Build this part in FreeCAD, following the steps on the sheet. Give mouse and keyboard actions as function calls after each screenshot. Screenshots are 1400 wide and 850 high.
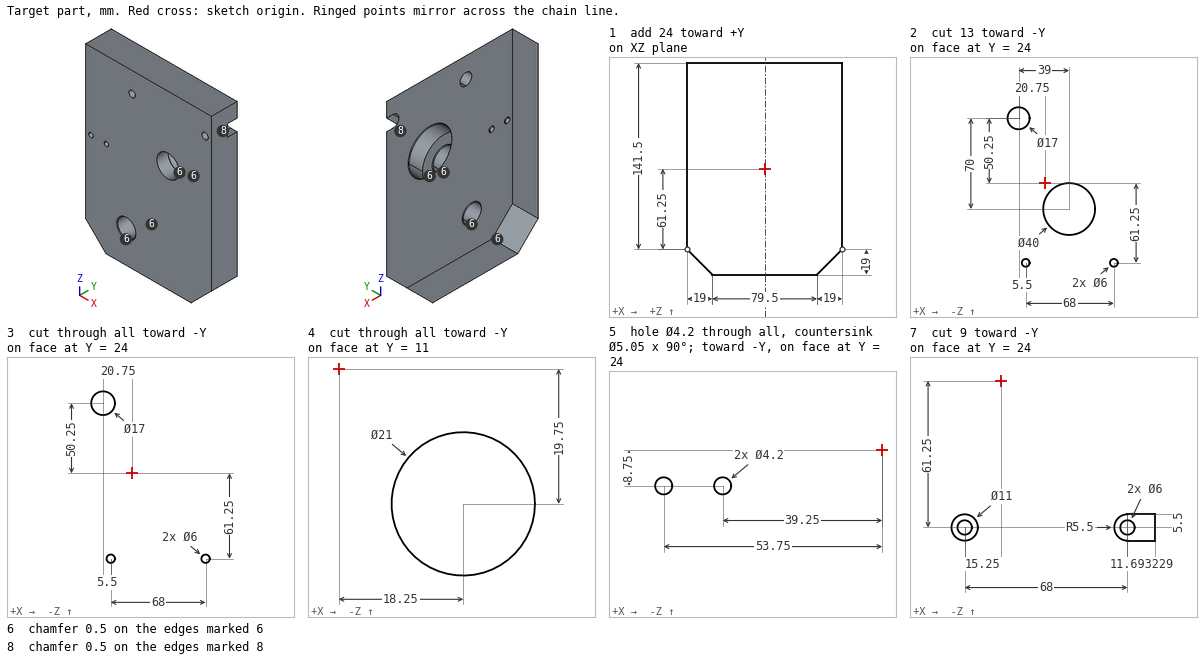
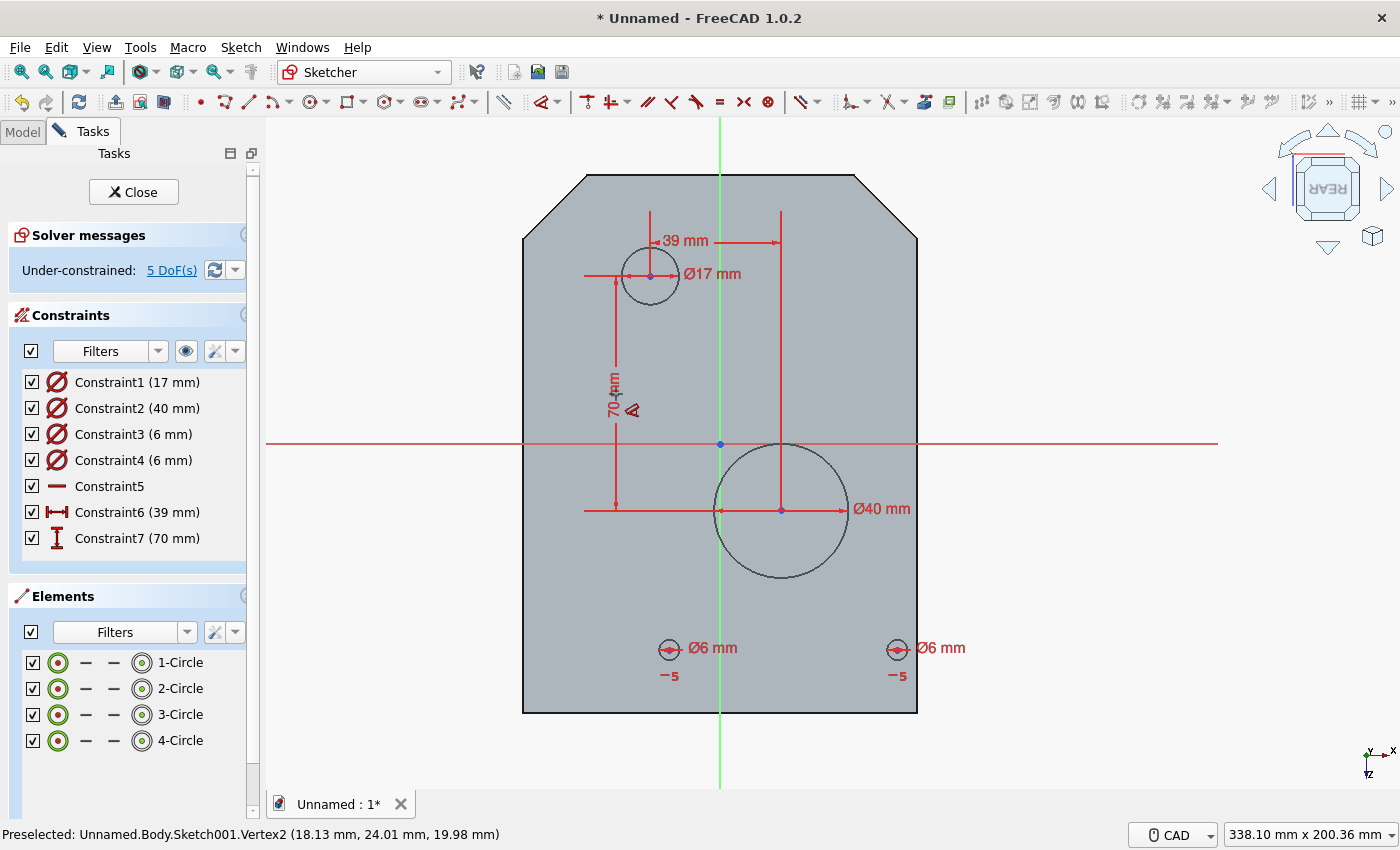
click(897, 650)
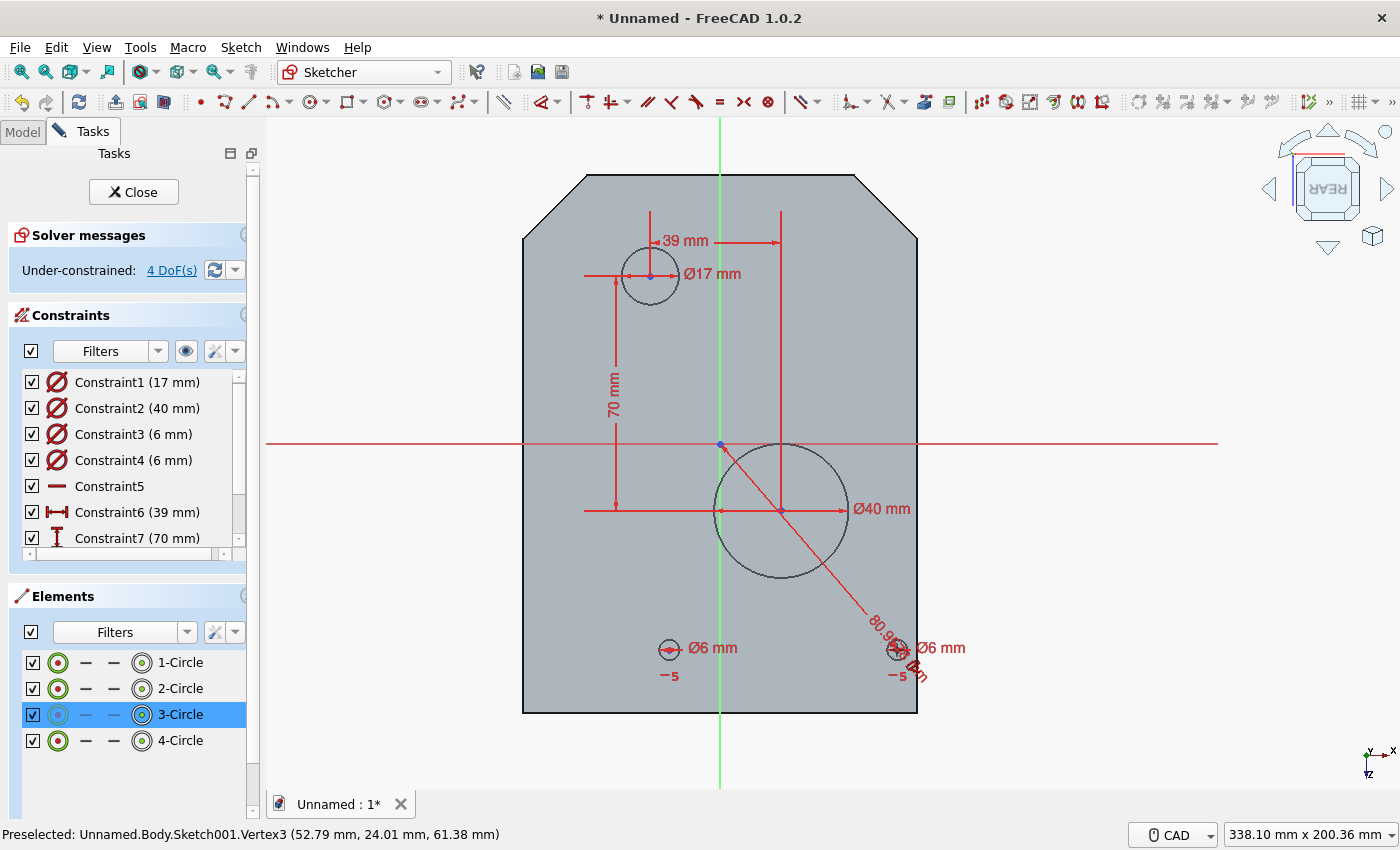
click(669, 650)
click(783, 684)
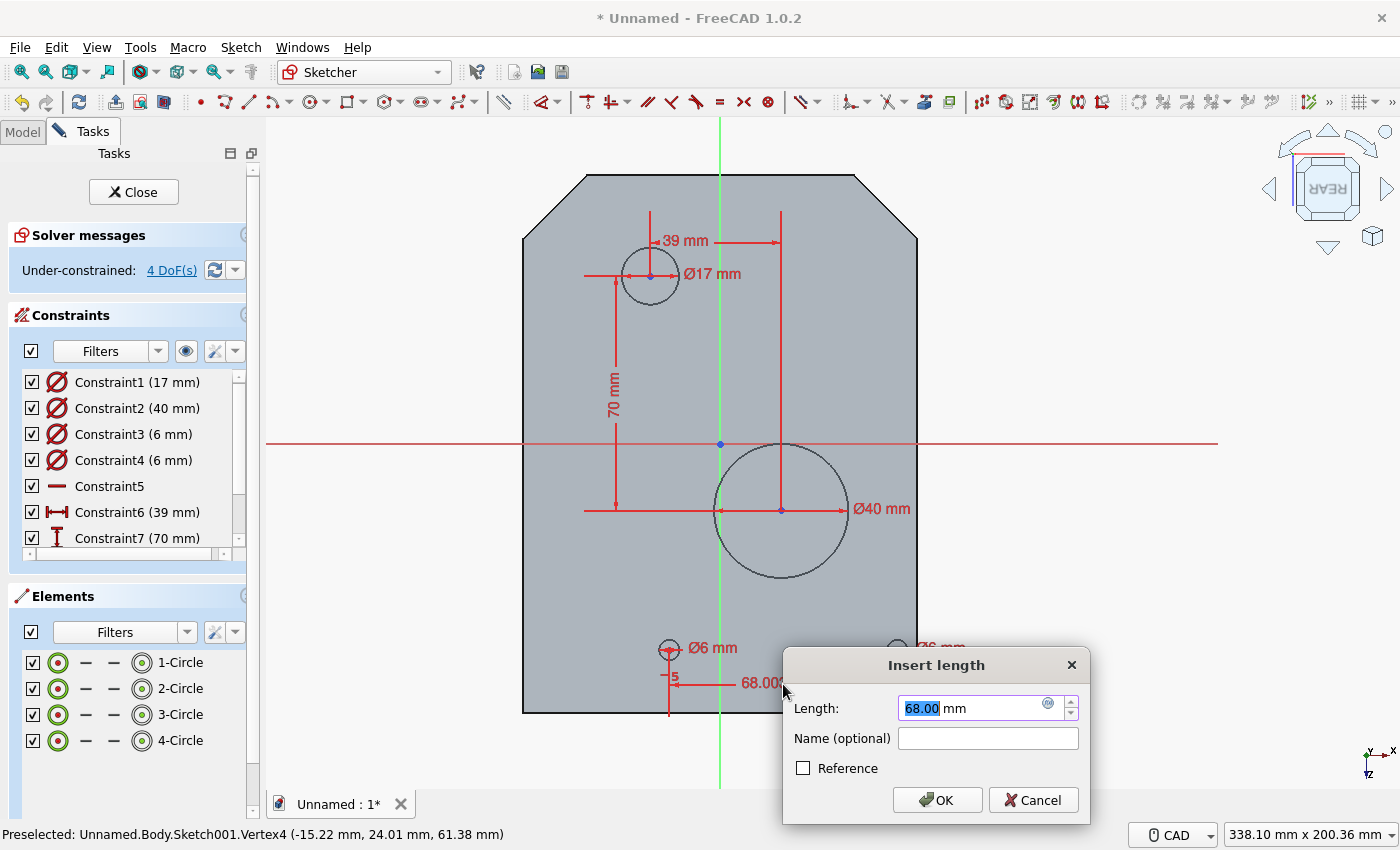
text(68)
key(Return)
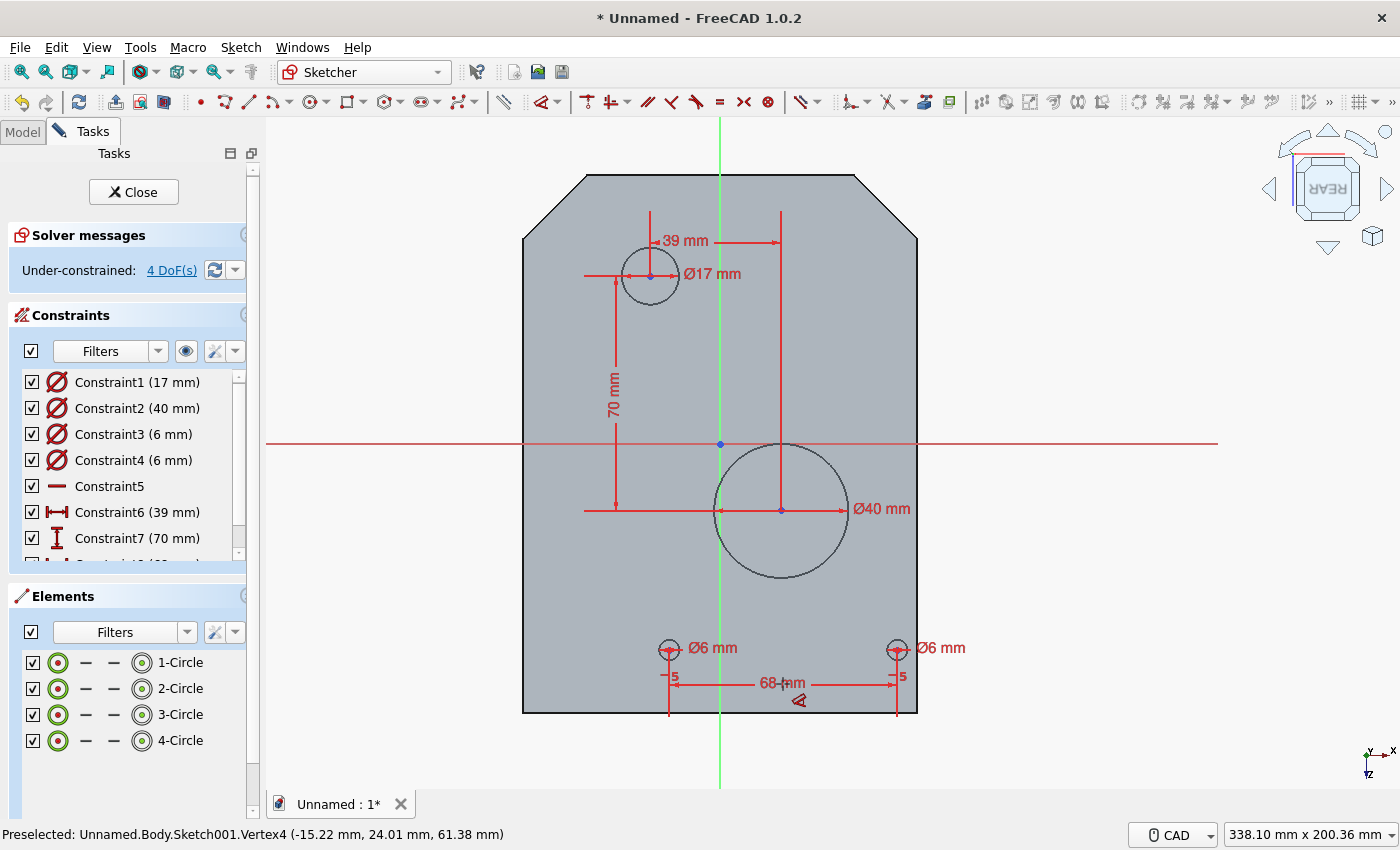
scroll(650, 276, up, 4)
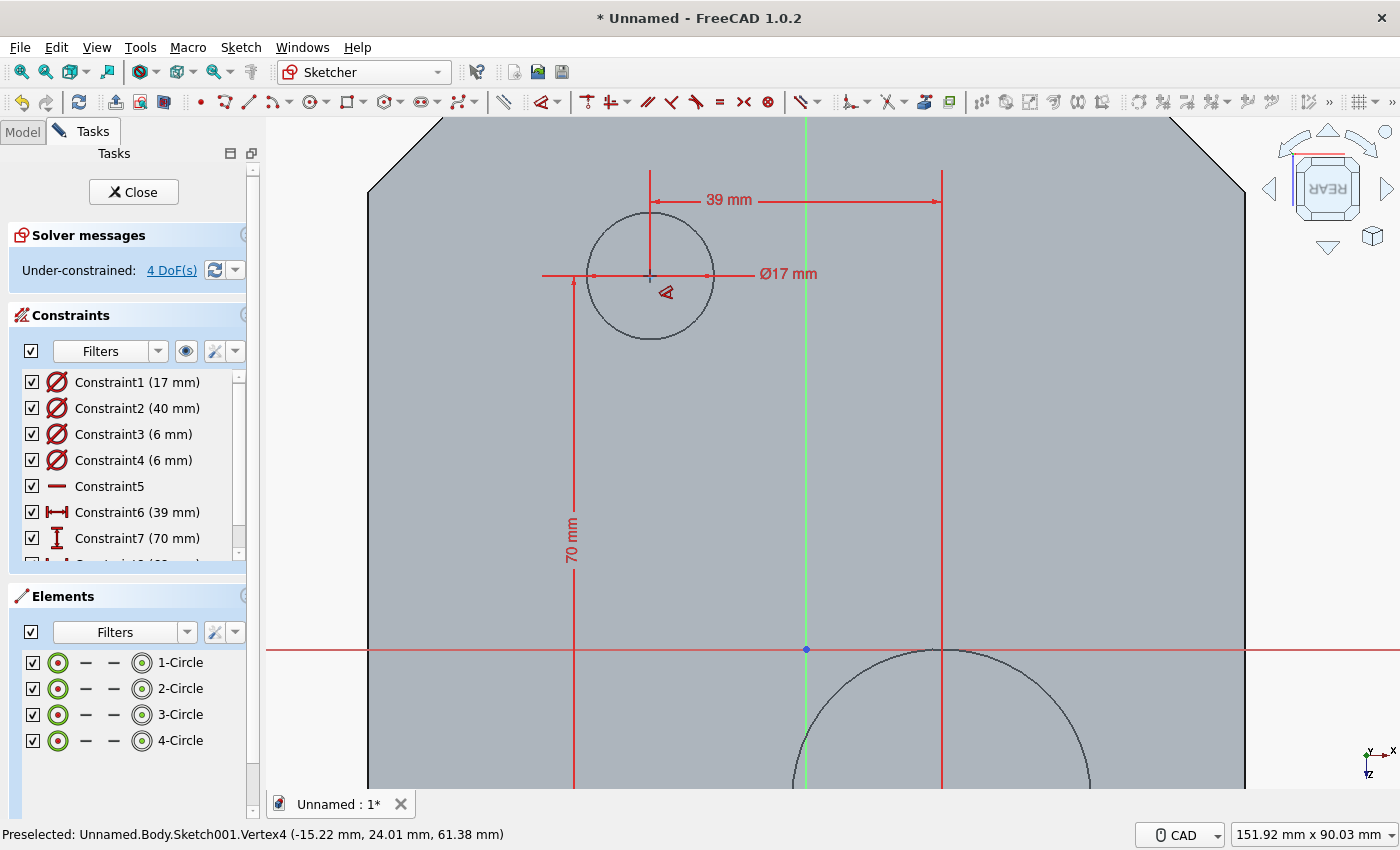
click(650, 276)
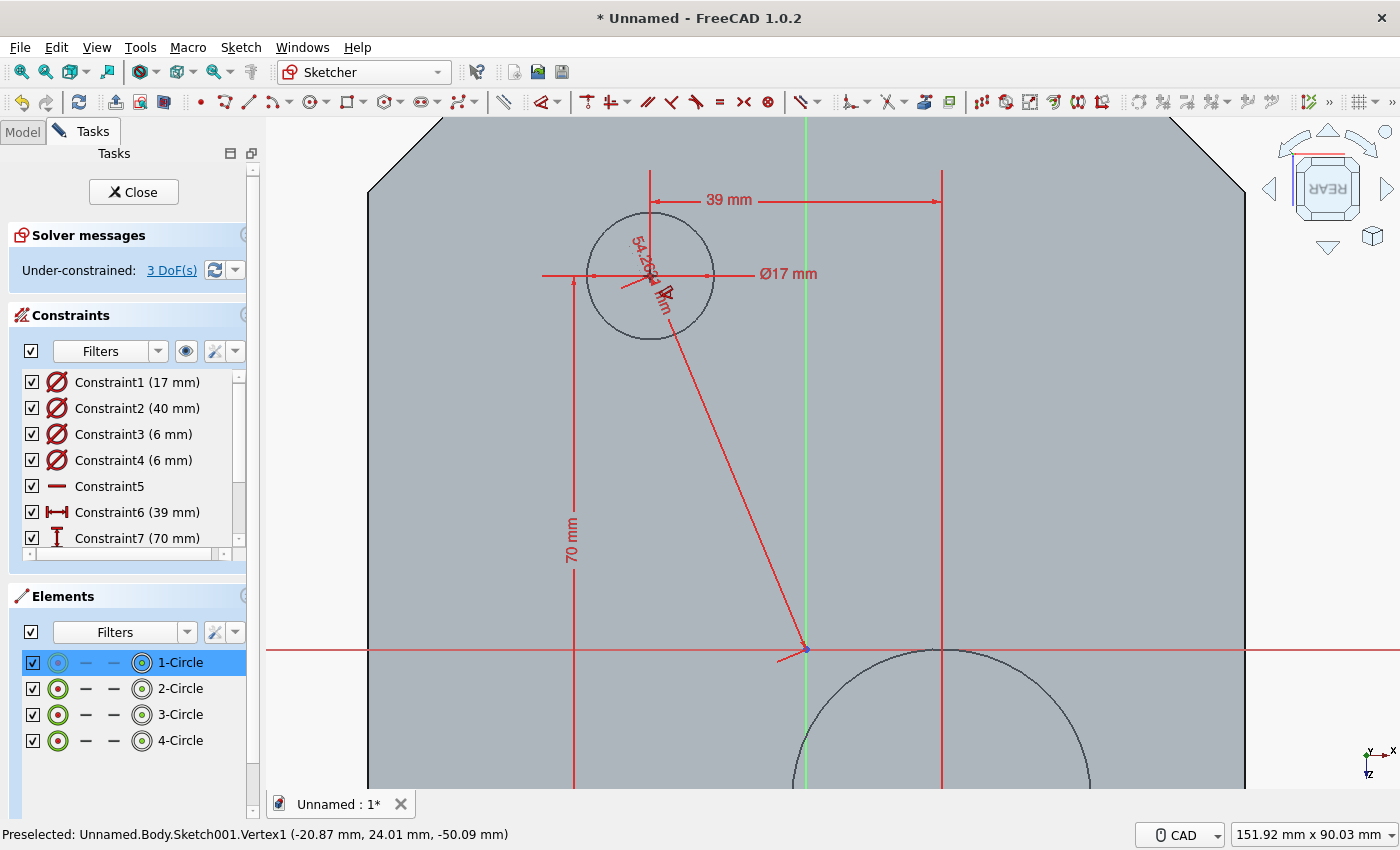
scroll(650, 276, down, 4)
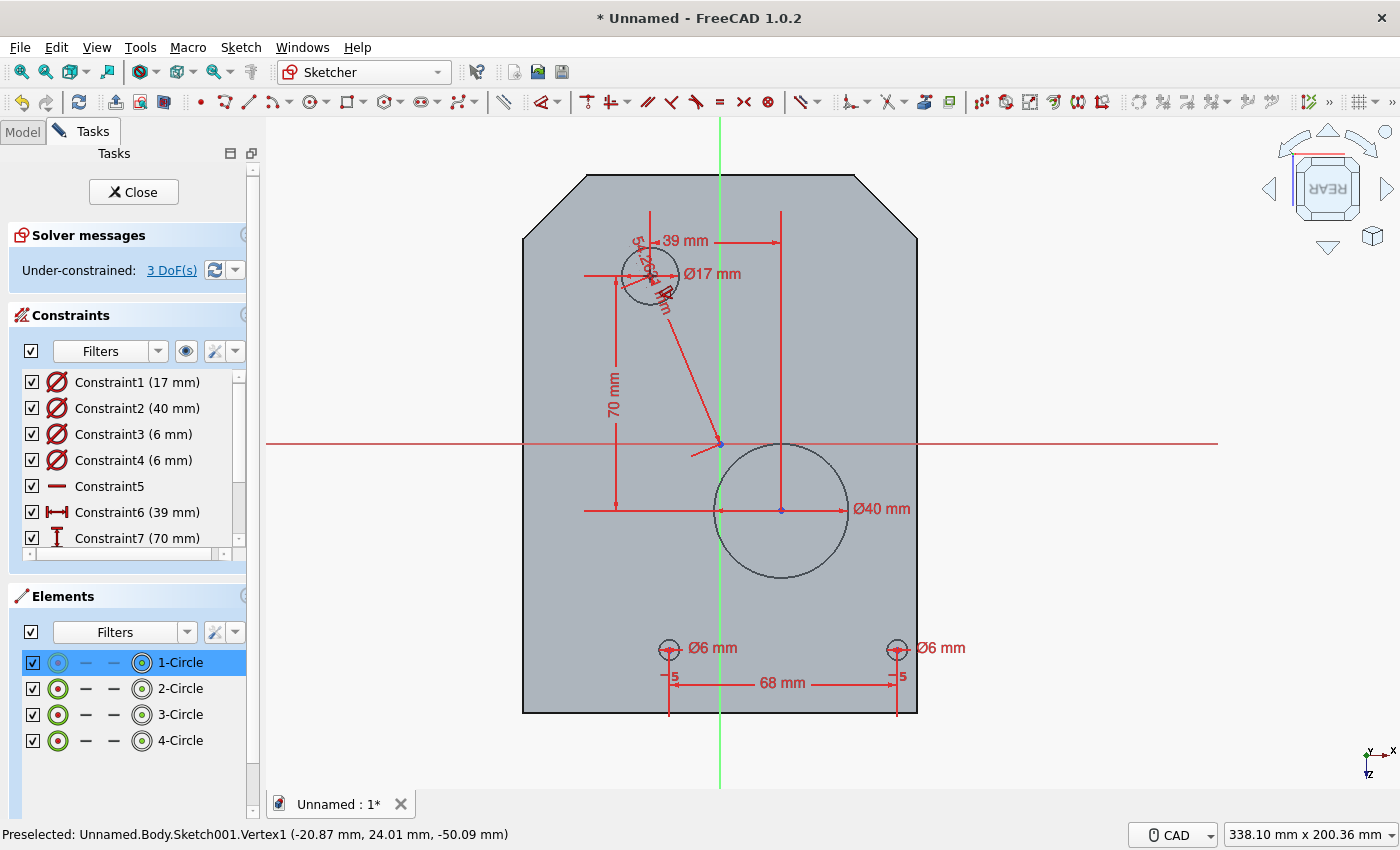
scroll(669, 650, up, 4)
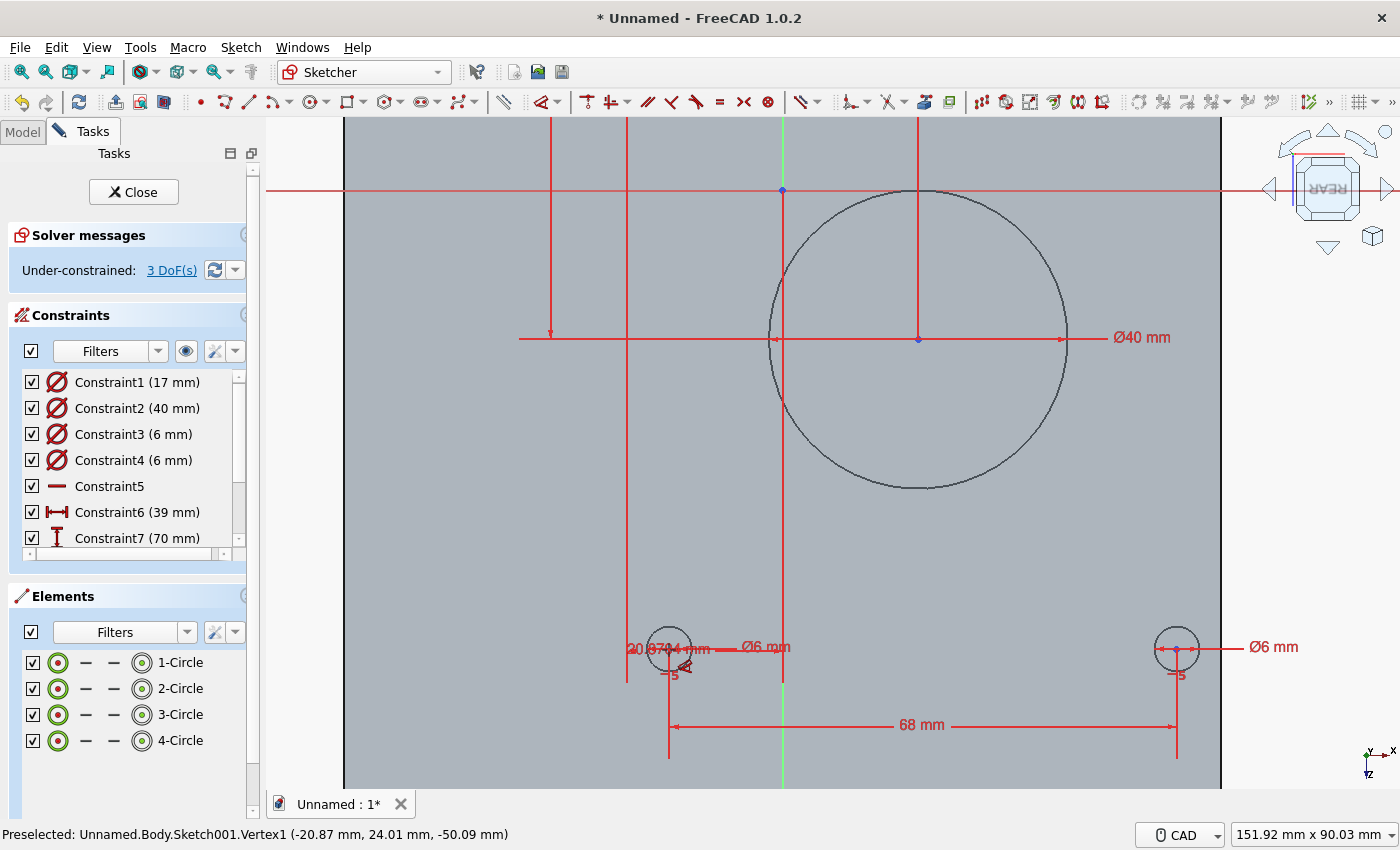
click(669, 649)
click(648, 683)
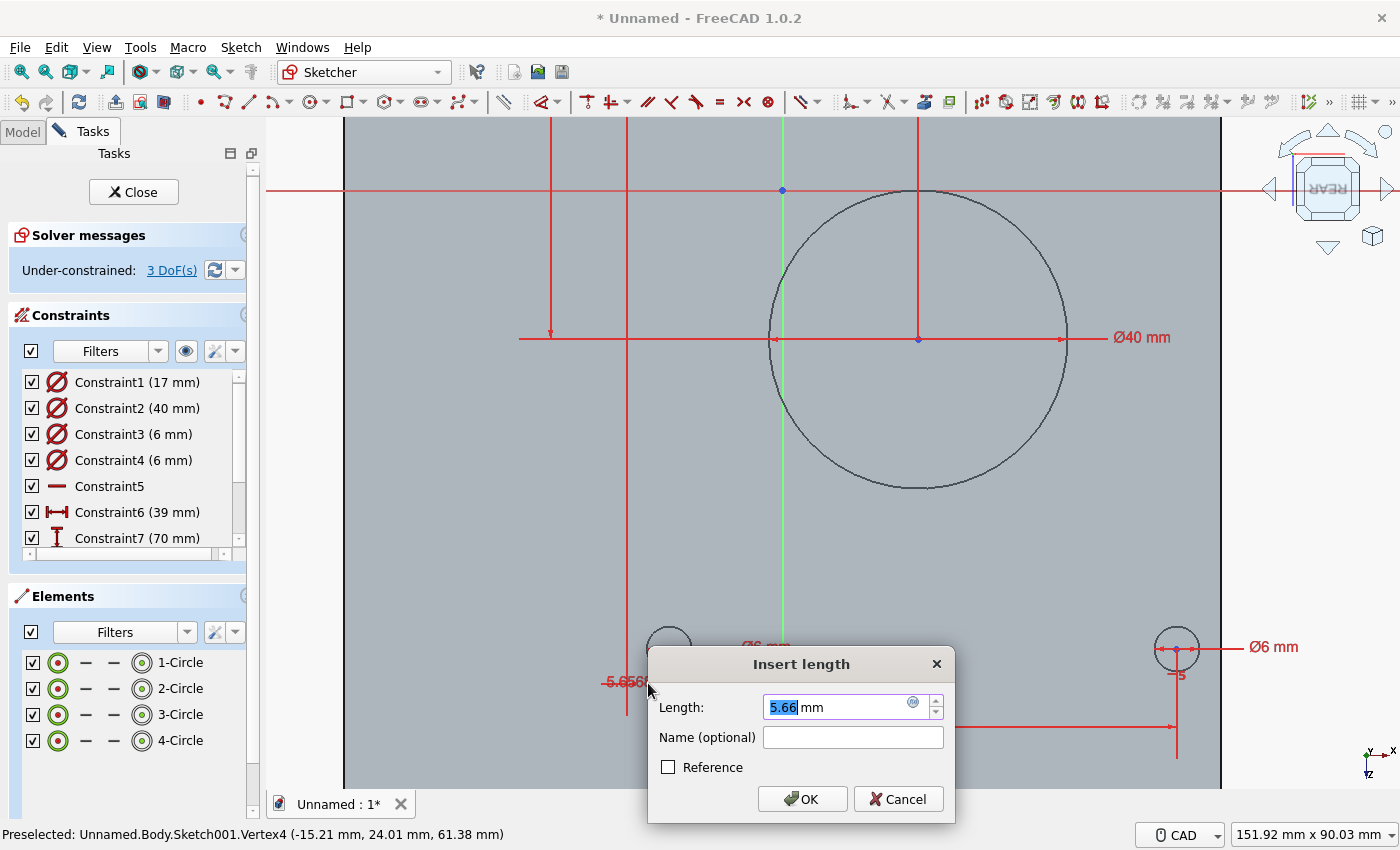
text(5.5)
key(Return)